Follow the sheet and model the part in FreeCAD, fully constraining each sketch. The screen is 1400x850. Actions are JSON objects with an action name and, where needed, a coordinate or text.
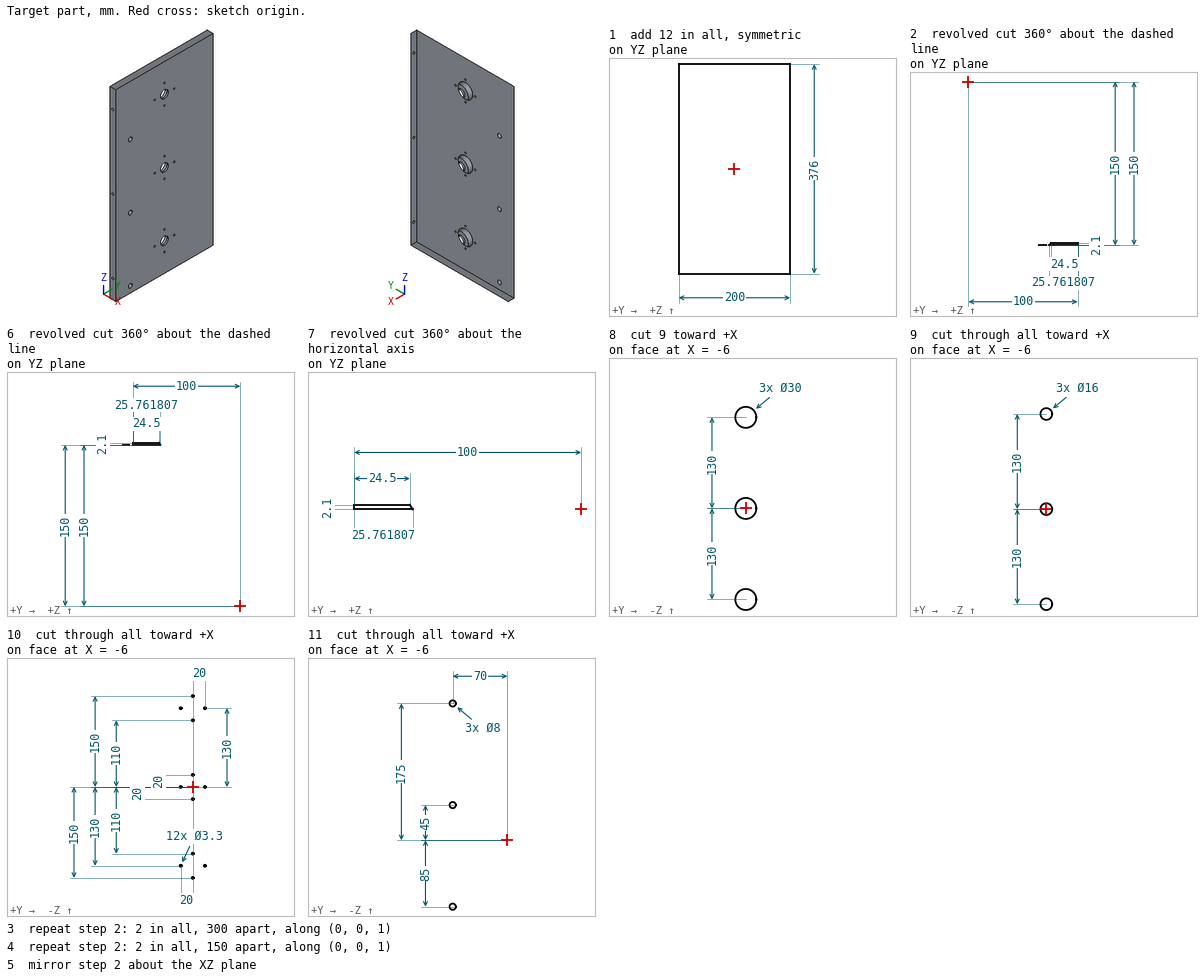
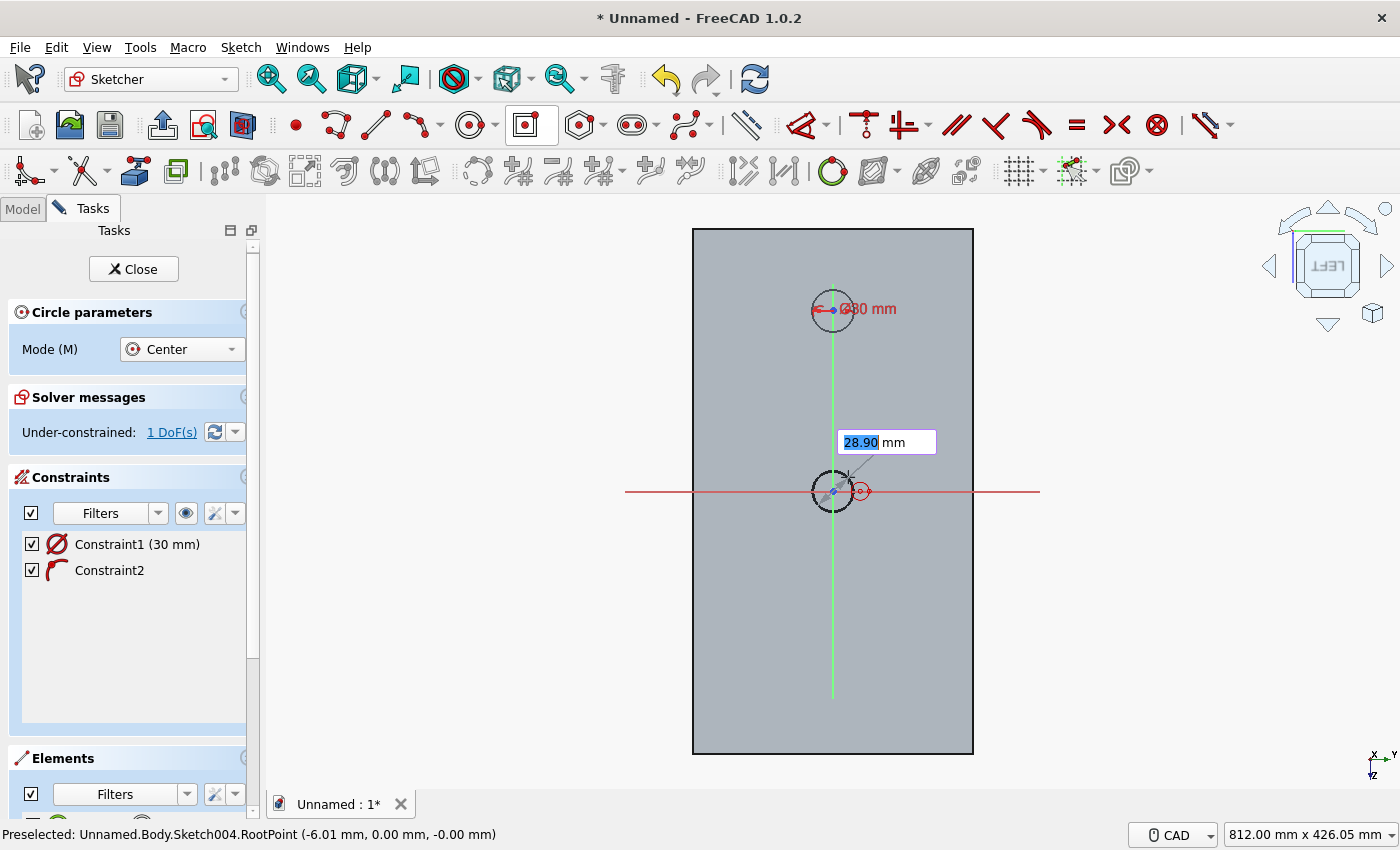
{"action": "type", "text": "30"}
{"action": "key", "text": "Return"}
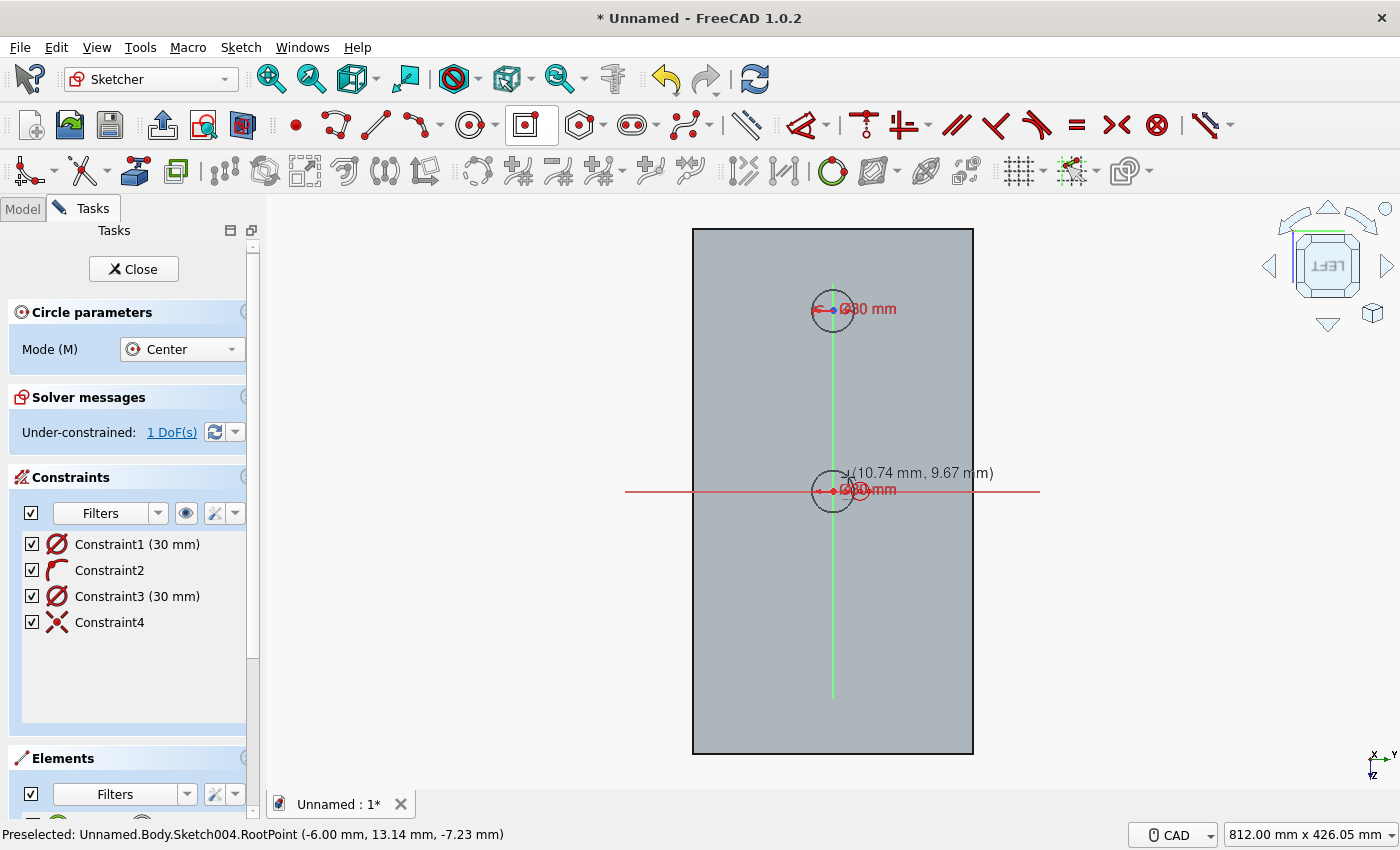
{"action": "left_click", "coordinate": [833, 673]}
{"action": "mouse_move", "coordinate": [848, 658]}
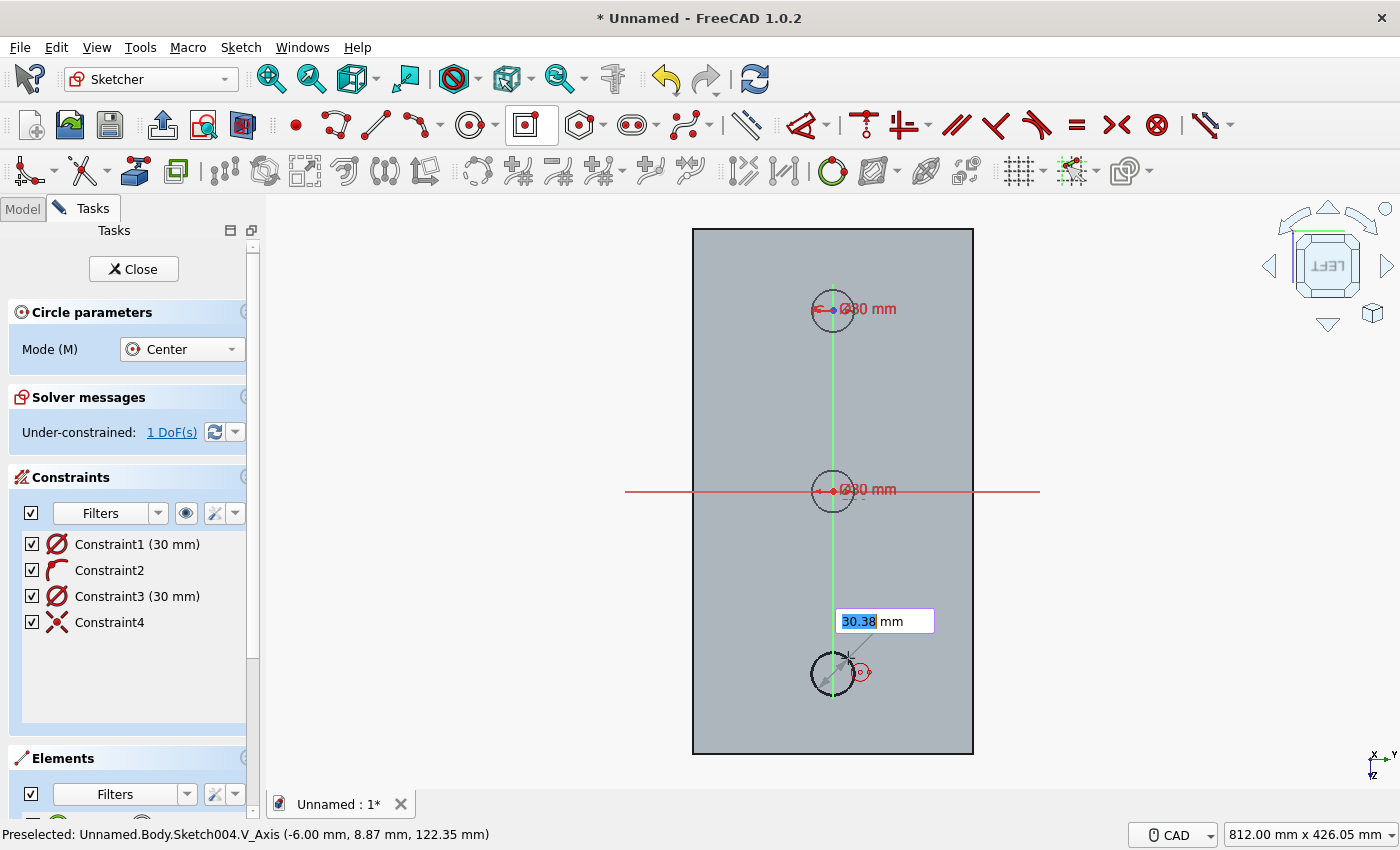
{"action": "type", "text": "30"}
{"action": "key", "text": "Return"}
{"action": "key", "text": "Escape"}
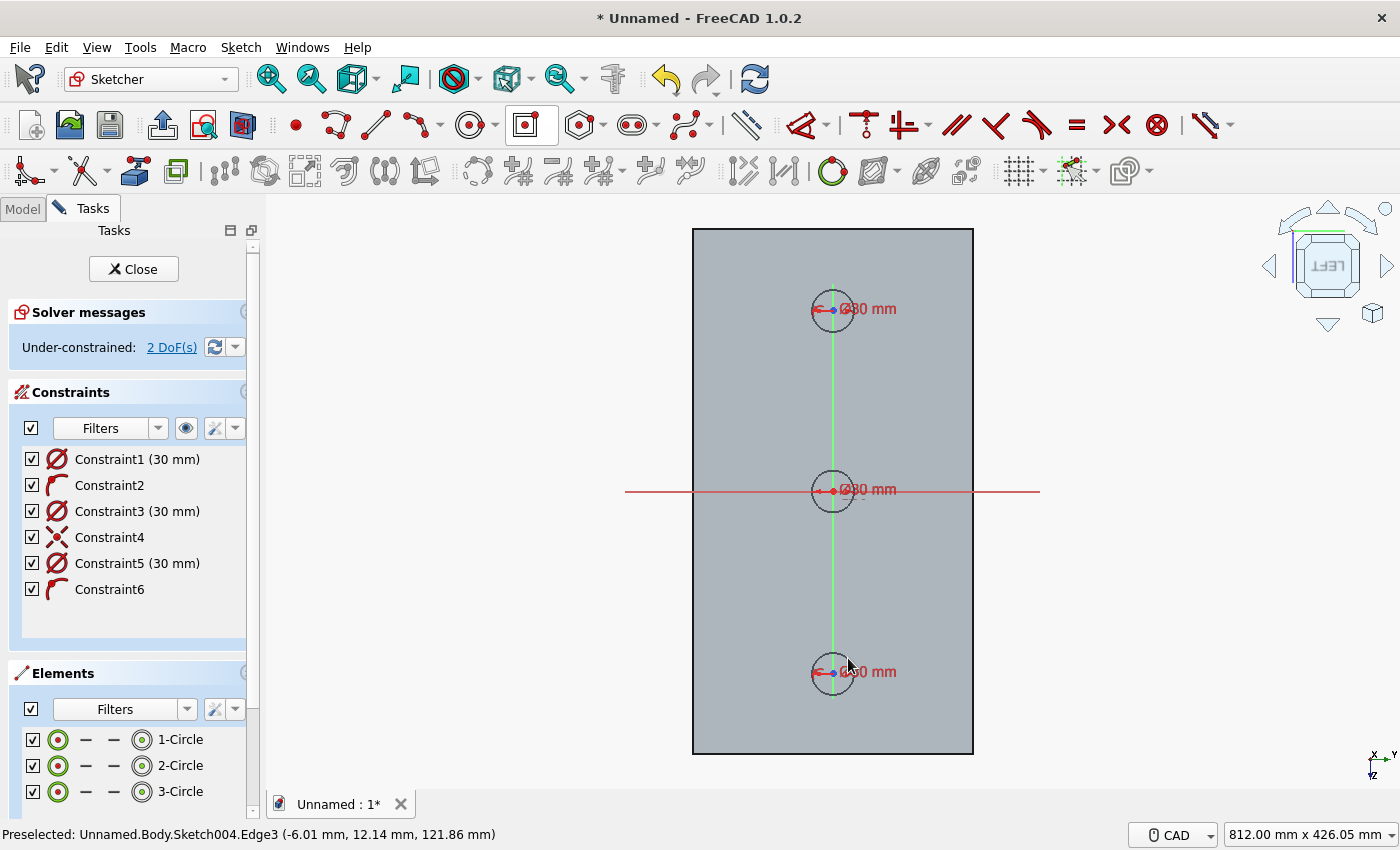
{"action": "left_click", "coordinate": [802, 126]}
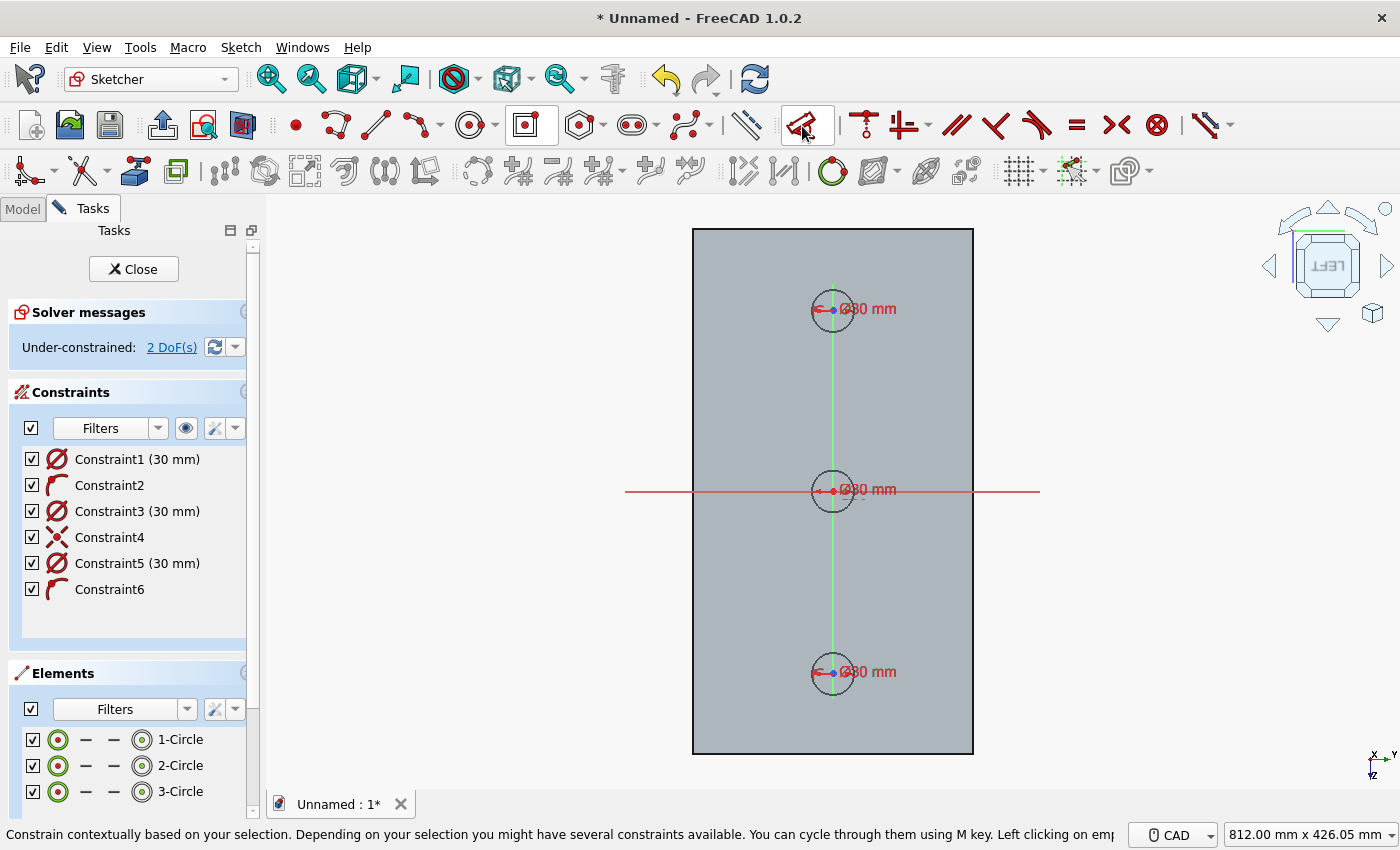
{"action": "left_click", "coordinate": [833, 311]}
{"action": "left_click", "coordinate": [867, 401]}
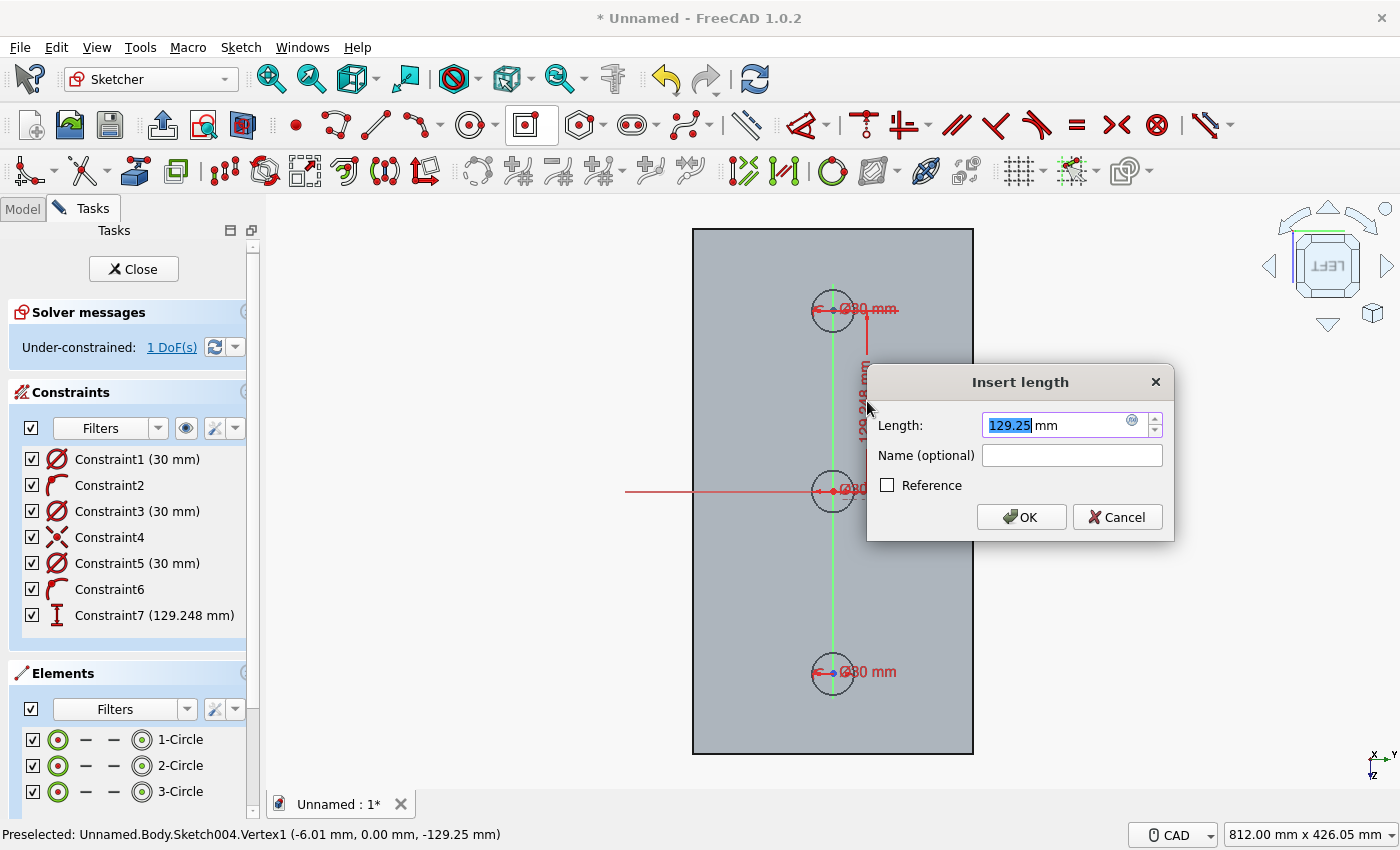
{"action": "type", "text": "130"}
{"action": "key", "text": "Return"}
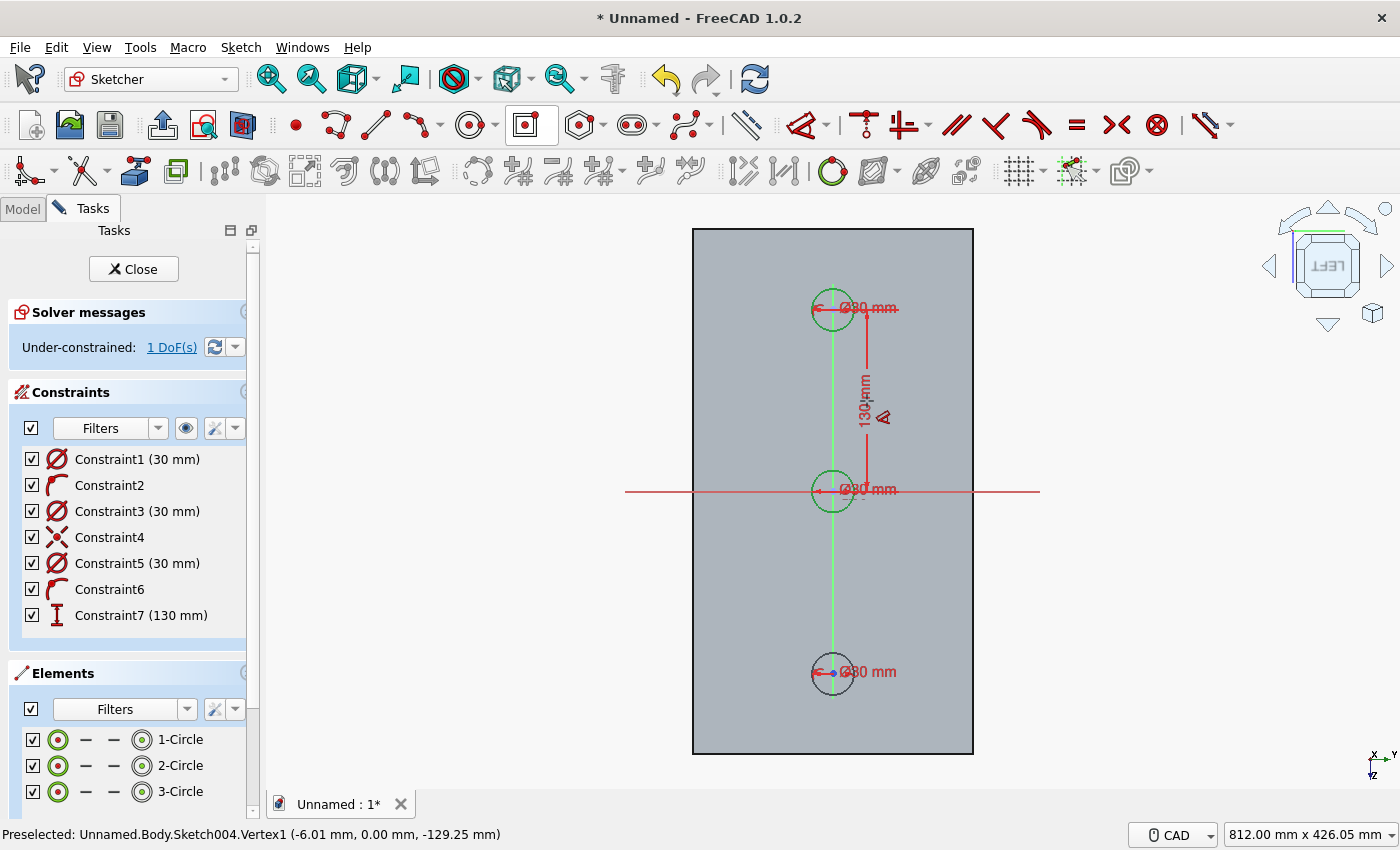
{"action": "left_click", "coordinate": [833, 674]}
{"action": "left_click", "coordinate": [867, 583]}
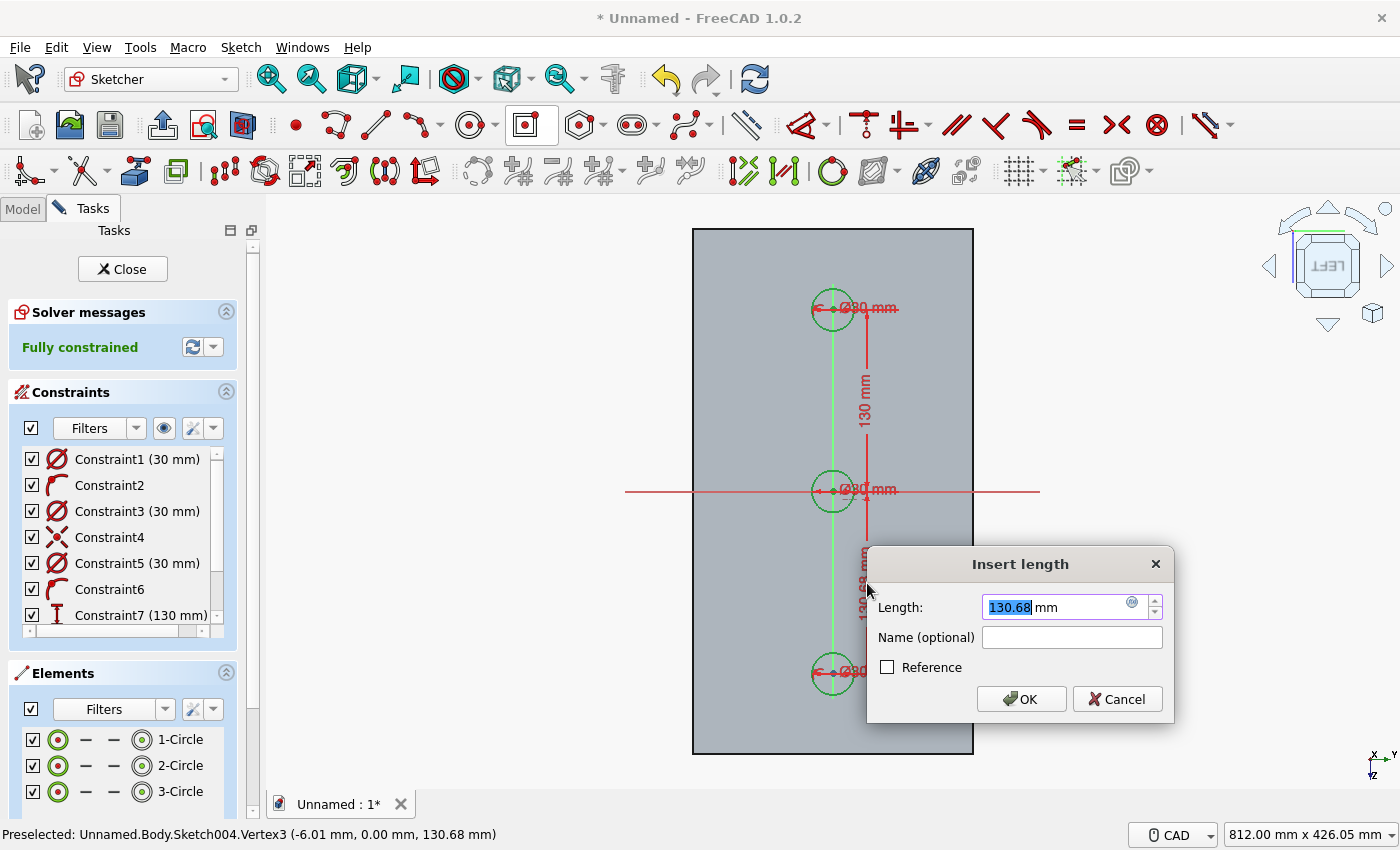
{"action": "type", "text": "130"}
{"action": "key", "text": "Return"}
{"action": "key", "text": "Escape"}